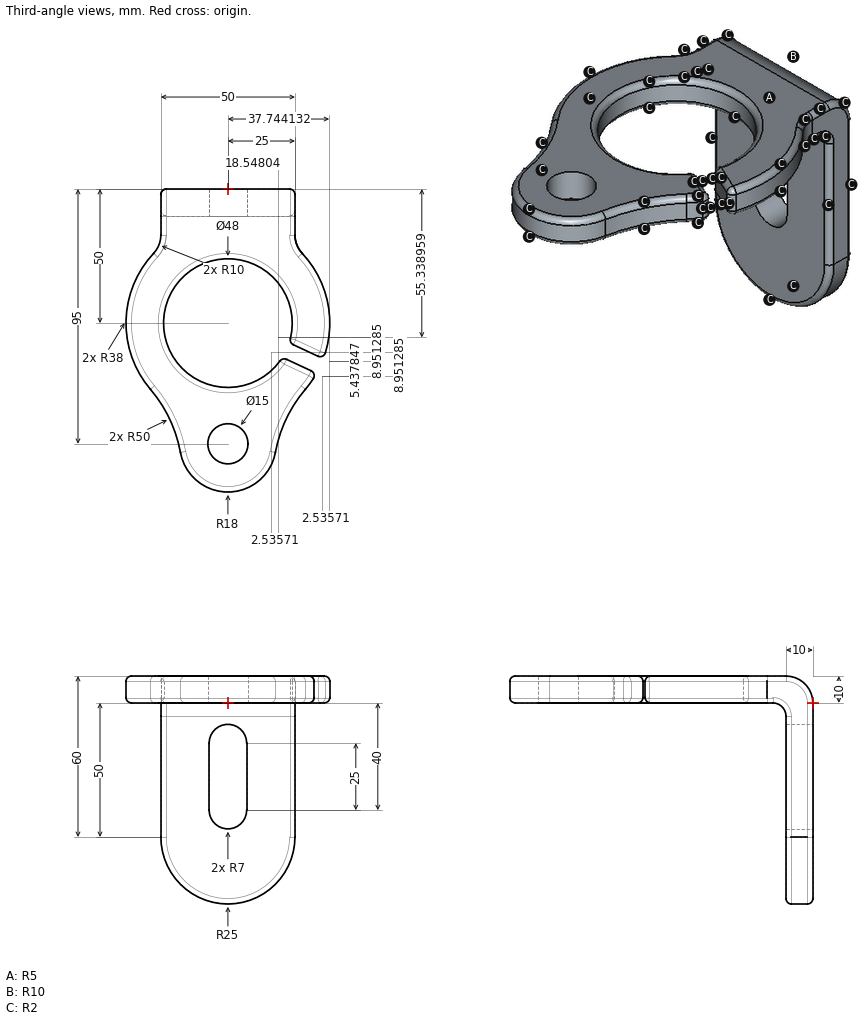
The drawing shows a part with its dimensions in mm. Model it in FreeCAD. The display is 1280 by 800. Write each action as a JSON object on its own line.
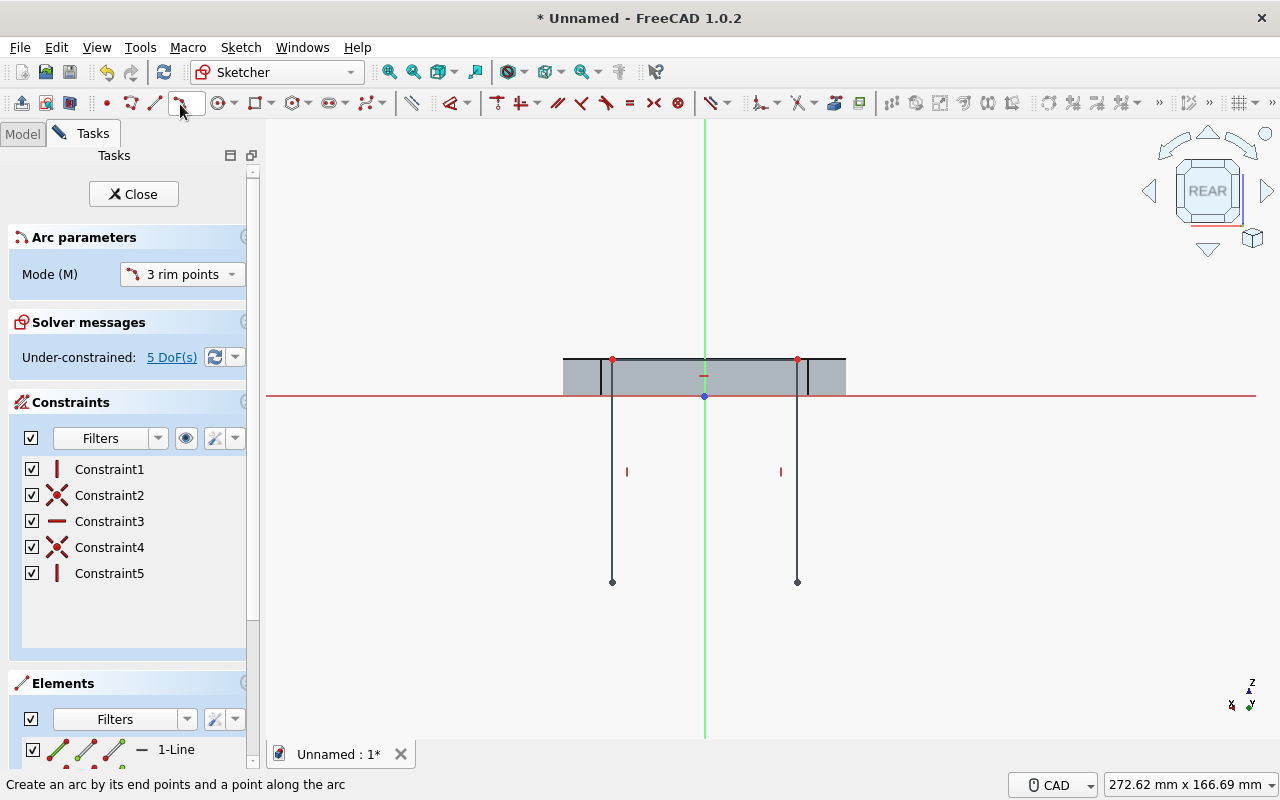
{"action": "left_click", "coordinate": [612, 583]}
{"action": "left_click", "coordinate": [797, 583]}
{"action": "left_click", "coordinate": [676, 671]}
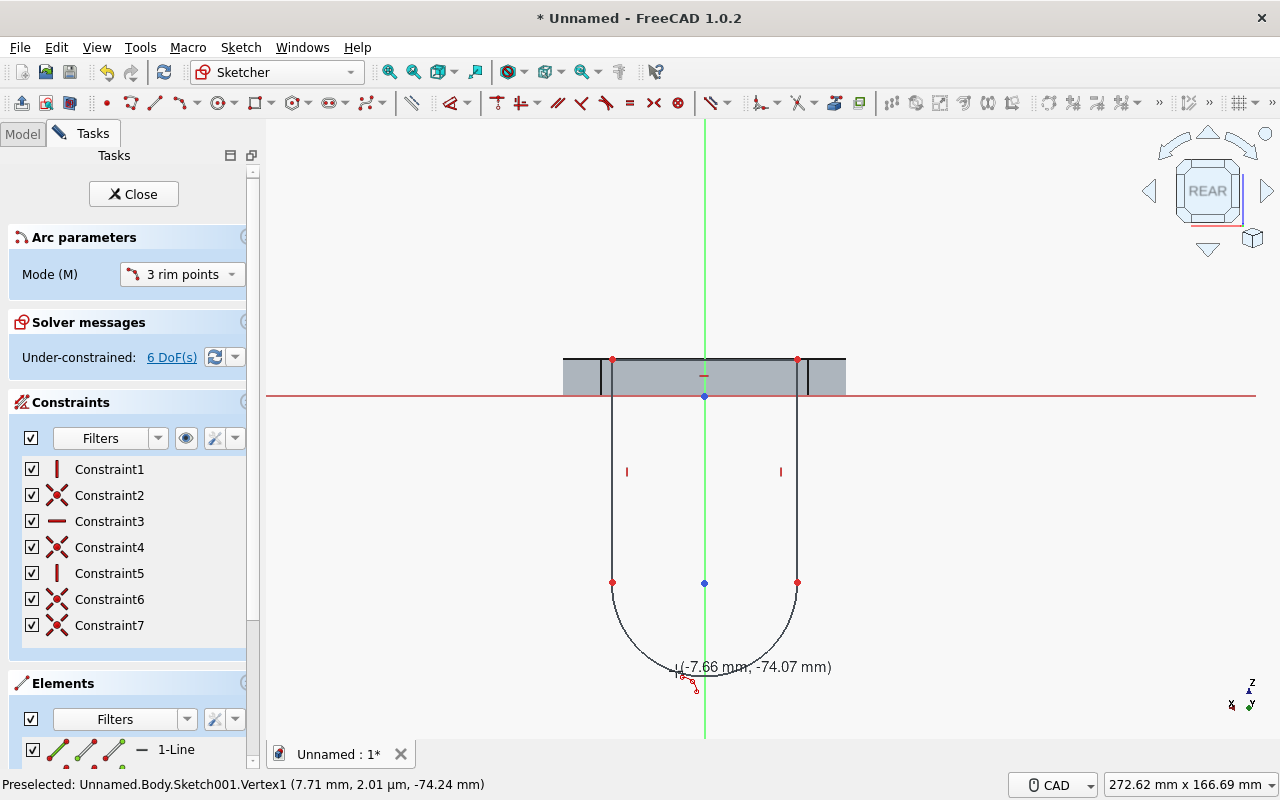
{"action": "left_click", "coordinate": [330, 104]}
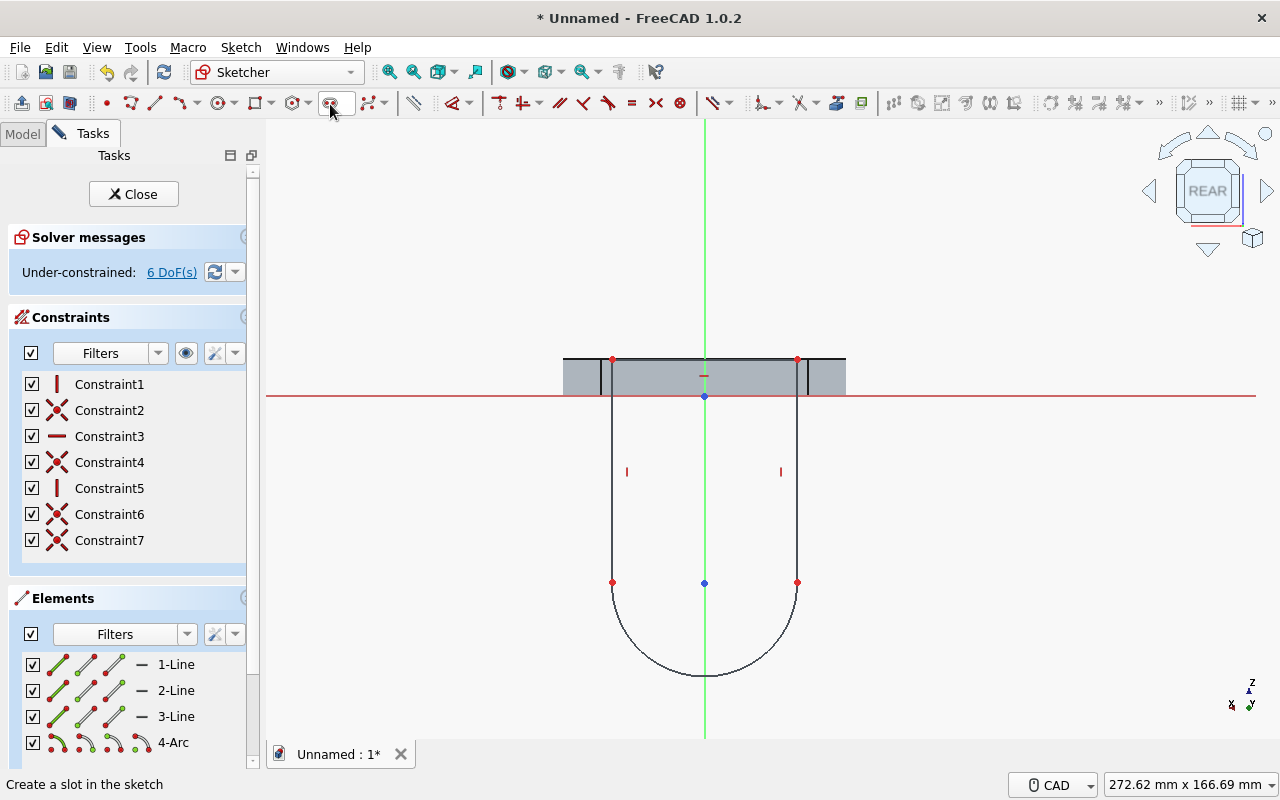
{"action": "left_click", "coordinate": [705, 545]}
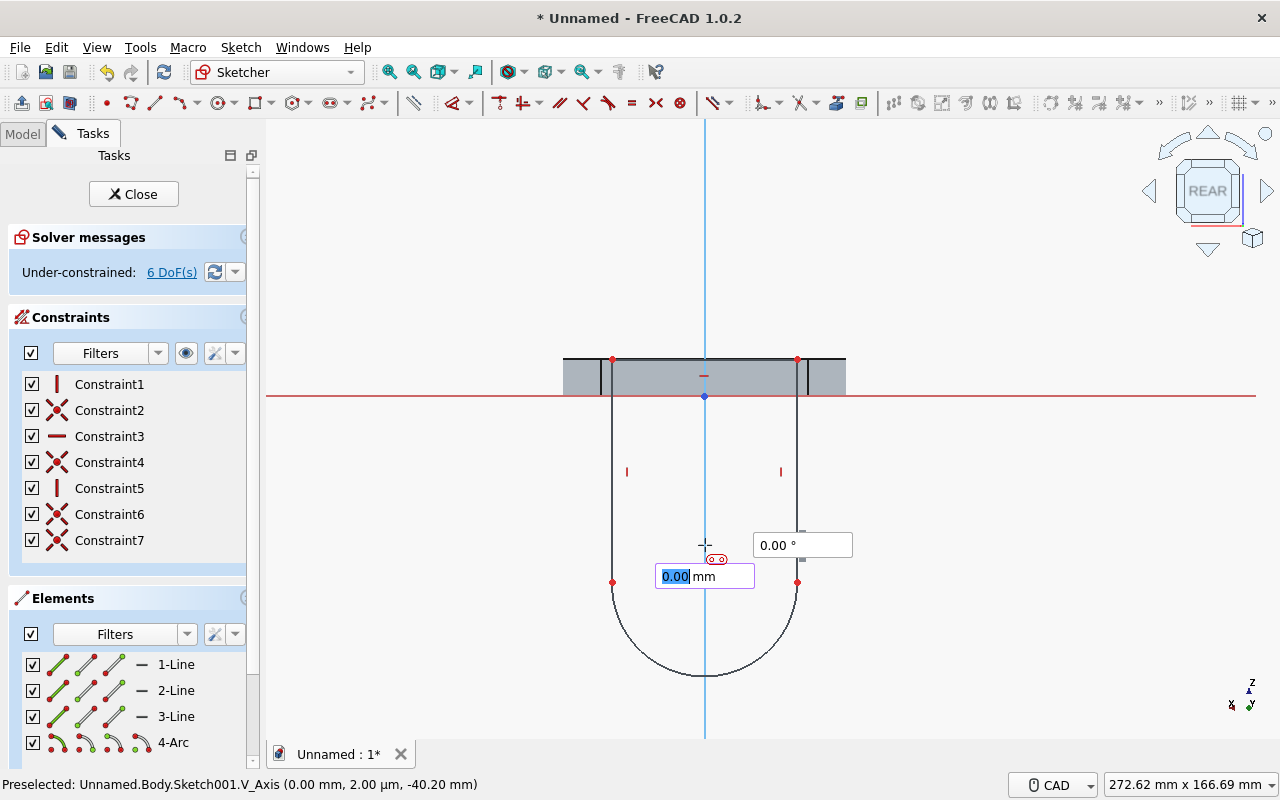
{"action": "left_click", "coordinate": [714, 452]}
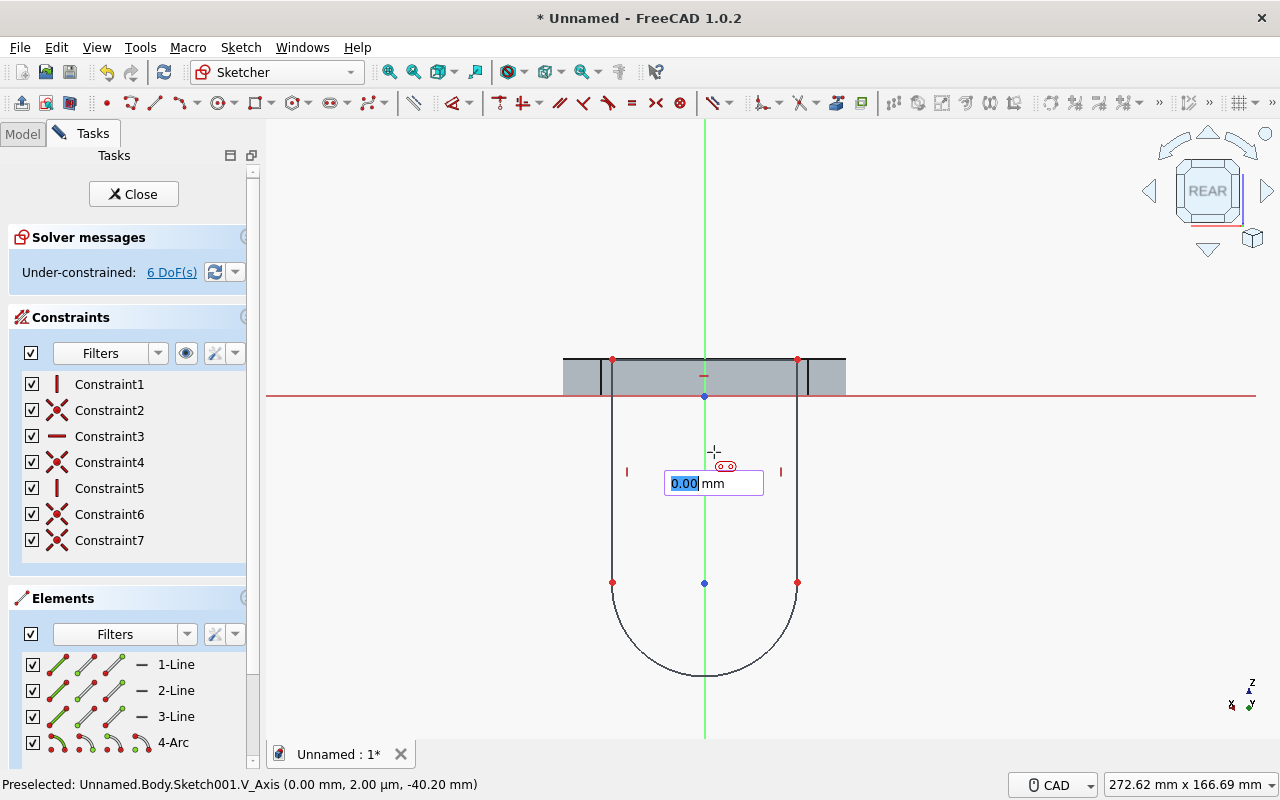
{"action": "left_click", "coordinate": [678, 499]}
{"action": "key", "text": "Escape"}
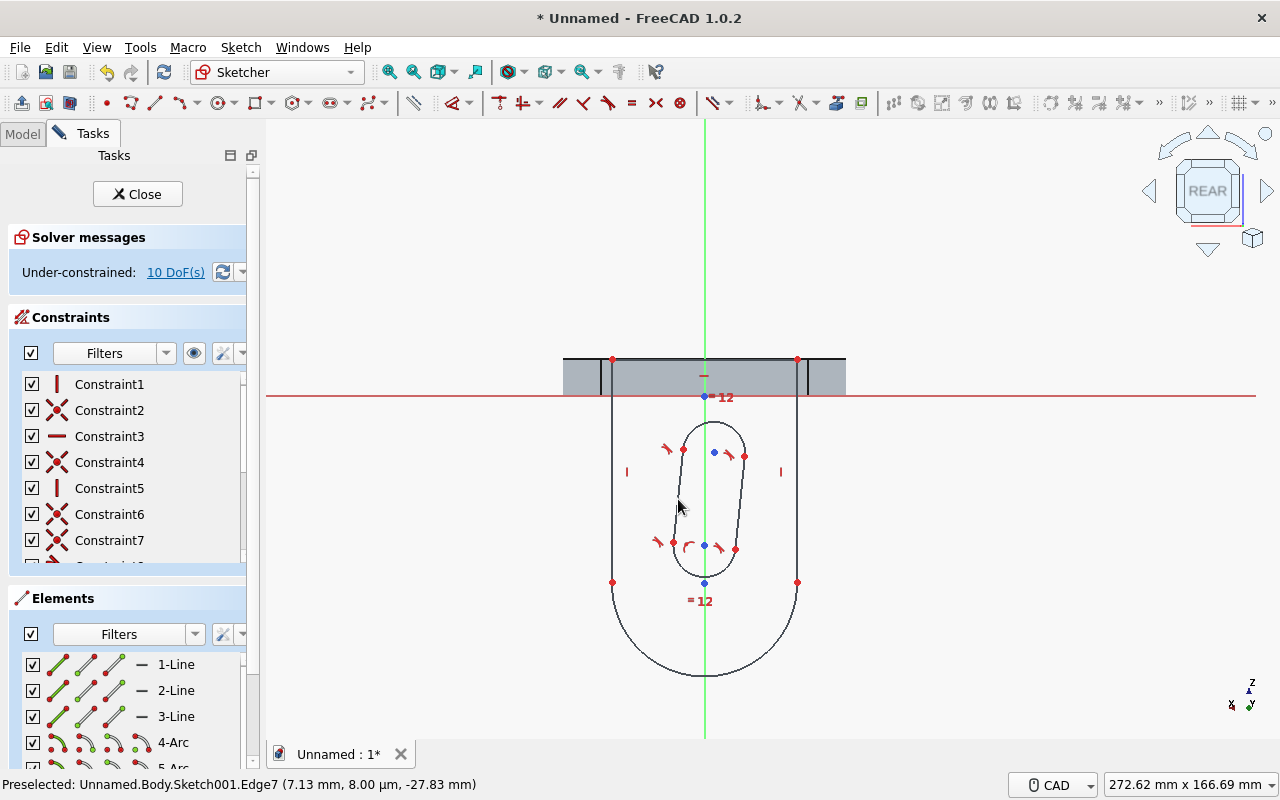
{"action": "left_click", "coordinate": [797, 516]}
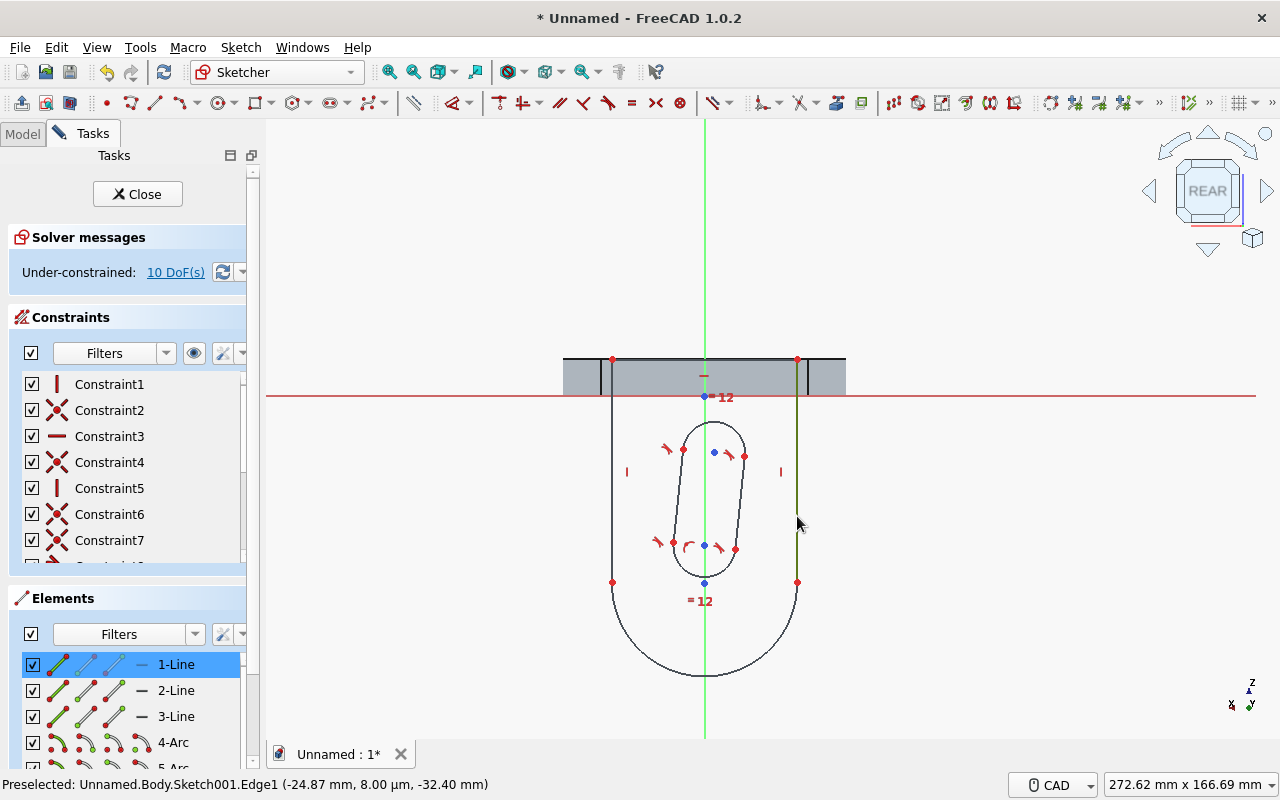
{"action": "left_click", "coordinate": [650, 659]}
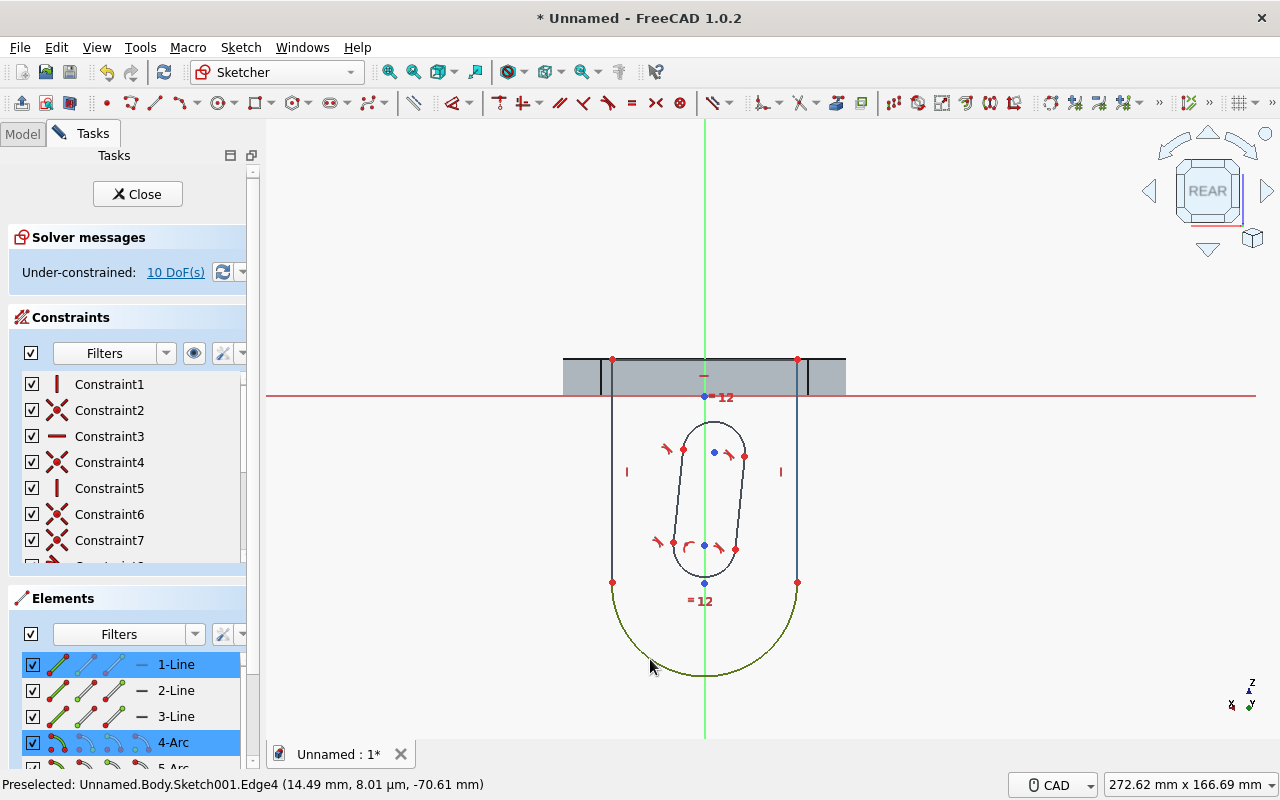
{"action": "left_click", "coordinate": [608, 104]}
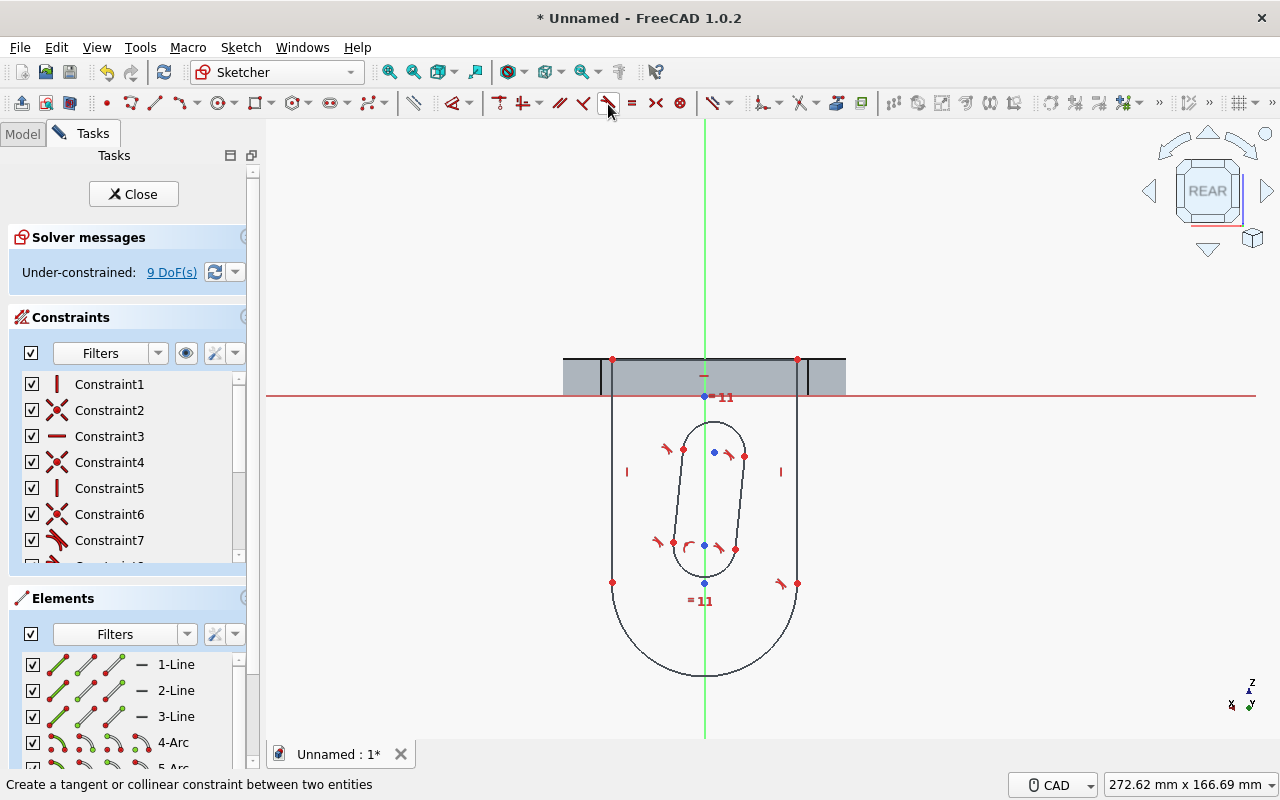
{"action": "left_click", "coordinate": [612, 427]}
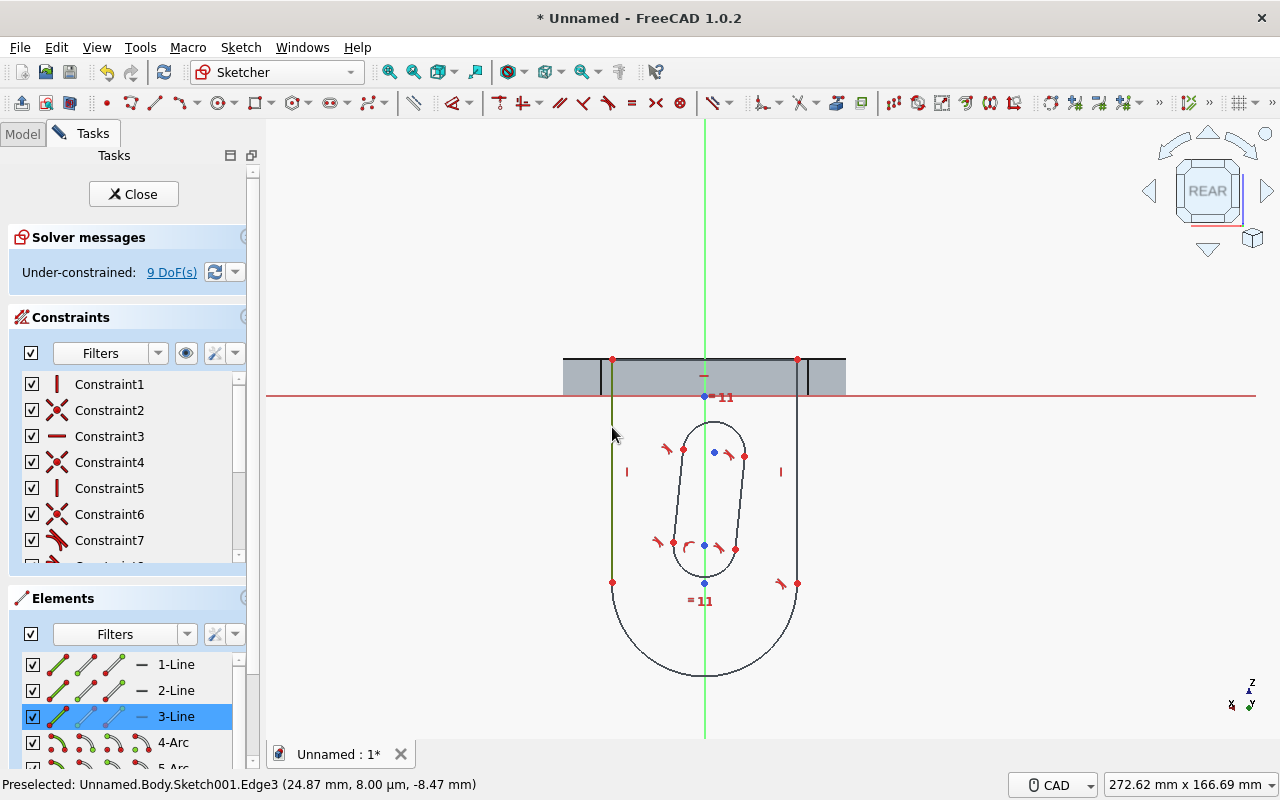
{"action": "left_click", "coordinate": [650, 658]}